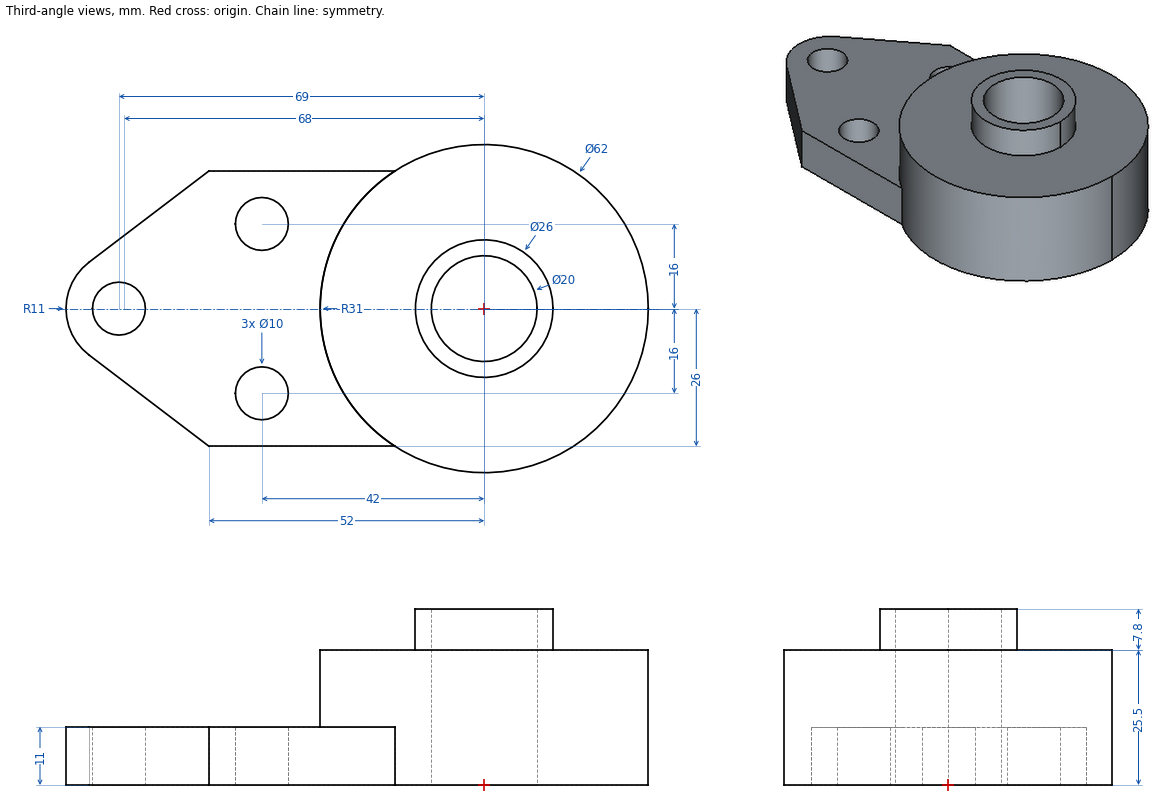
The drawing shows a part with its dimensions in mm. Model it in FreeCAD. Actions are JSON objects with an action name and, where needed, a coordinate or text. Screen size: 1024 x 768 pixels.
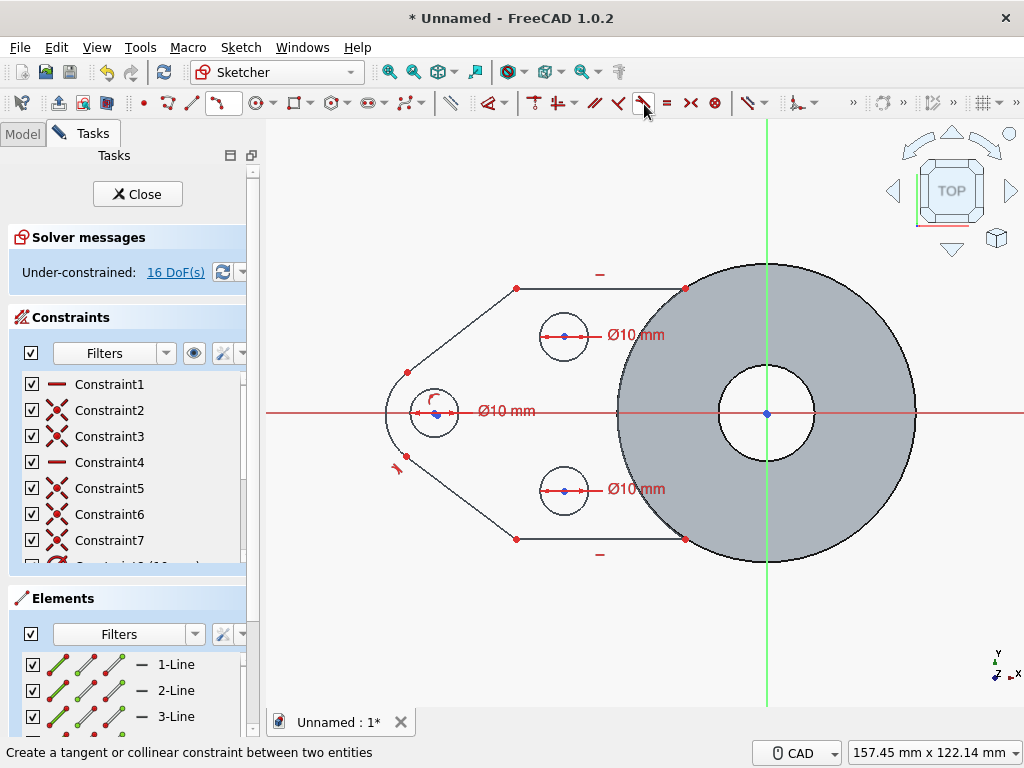
{"action": "left_click", "coordinate": [440, 348]}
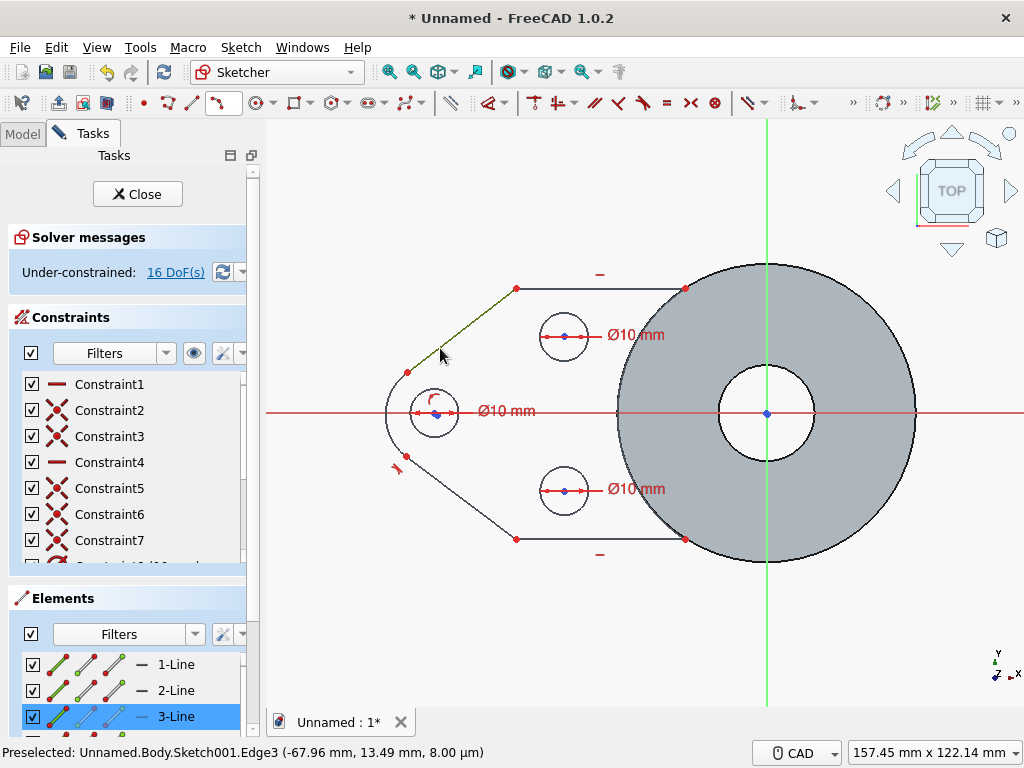
{"action": "left_click", "coordinate": [390, 395]}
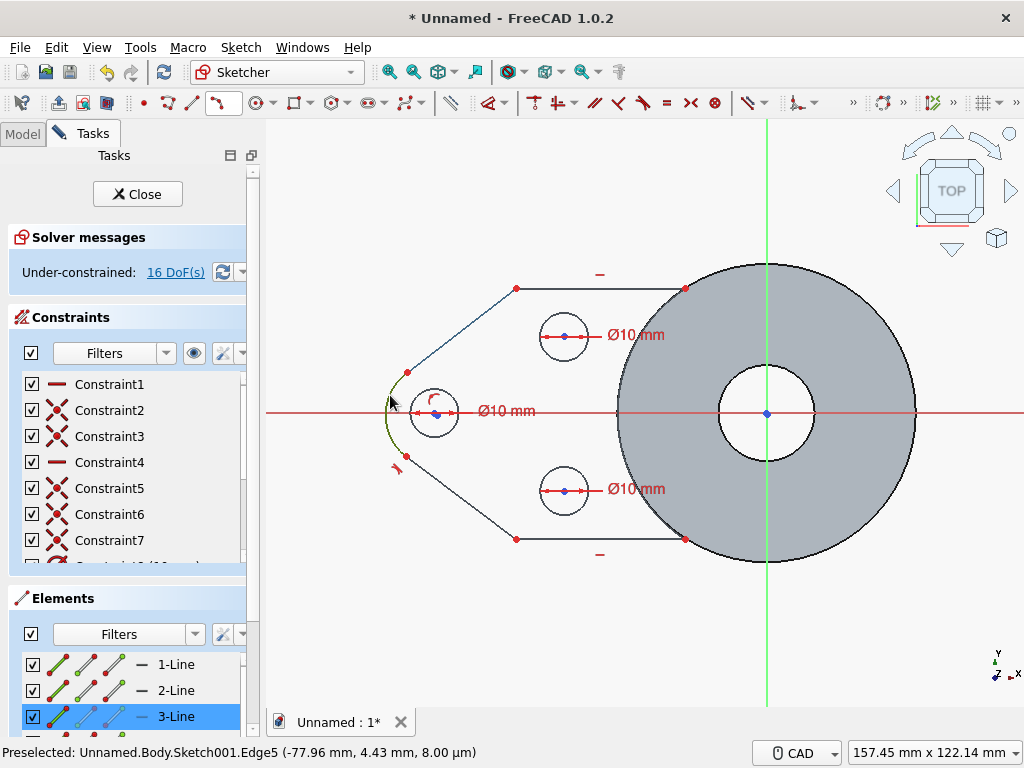
{"action": "left_click", "coordinate": [644, 104]}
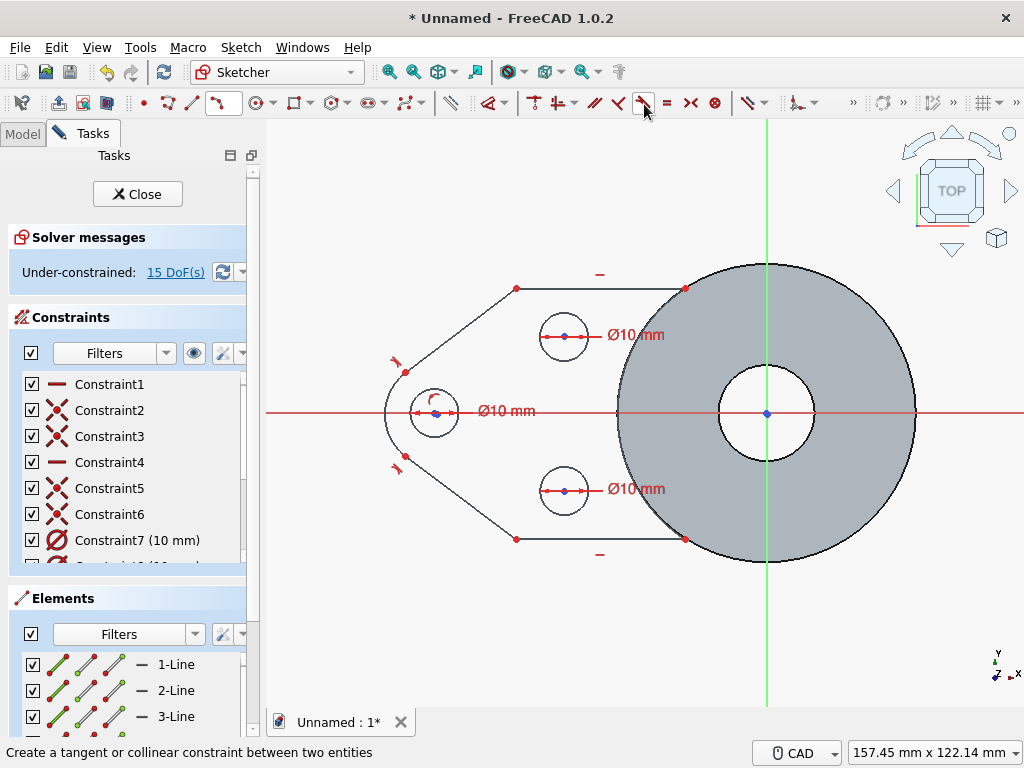
{"action": "scroll", "coordinate": [767, 414], "scroll_direction": "up", "scroll_amount": 3}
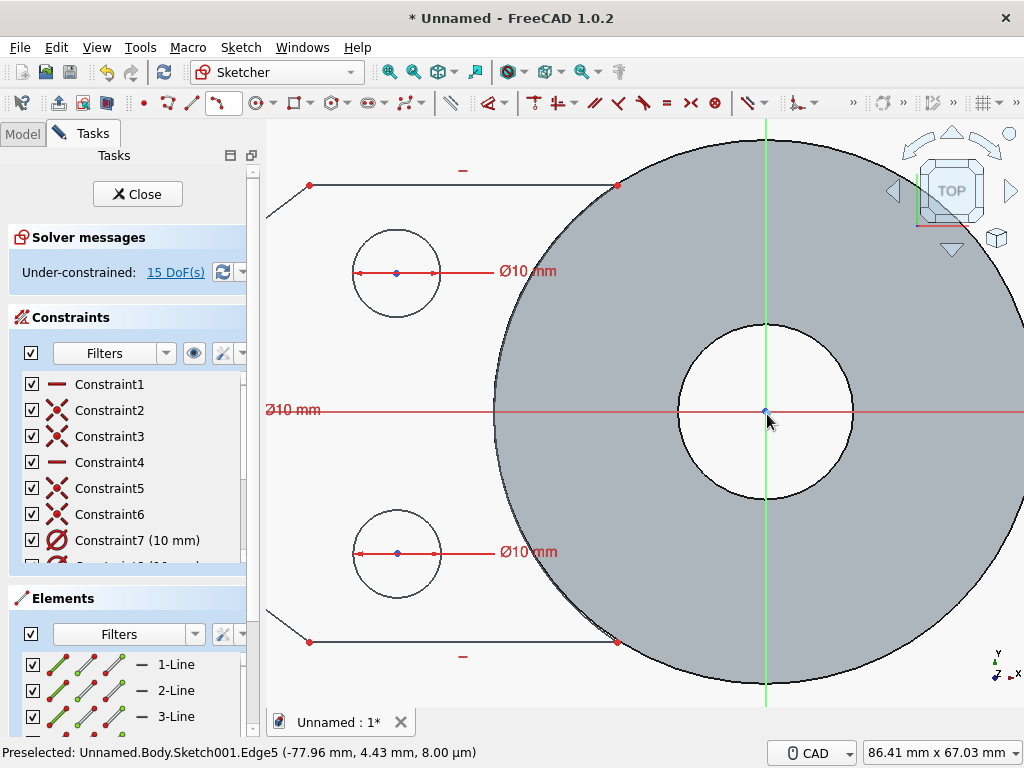
{"action": "left_click_drag", "start_coordinate": [756, 402], "coordinate": [778, 424]}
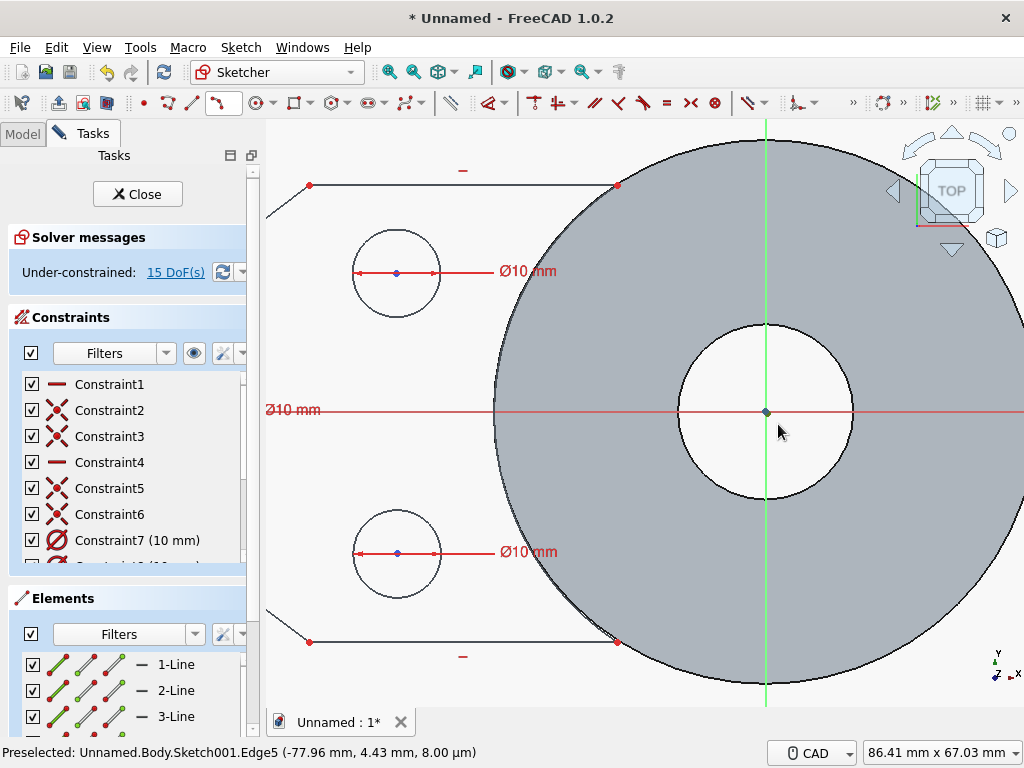
{"action": "key", "text": "c"}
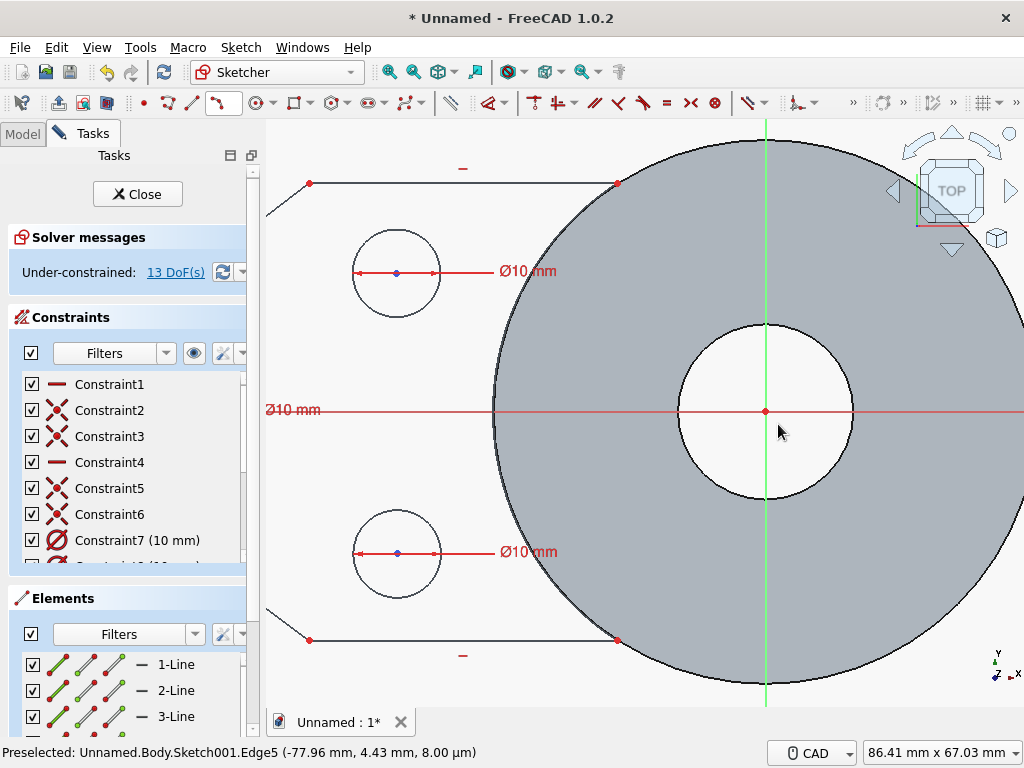
{"action": "scroll", "coordinate": [768, 414], "scroll_direction": "down", "scroll_amount": 3}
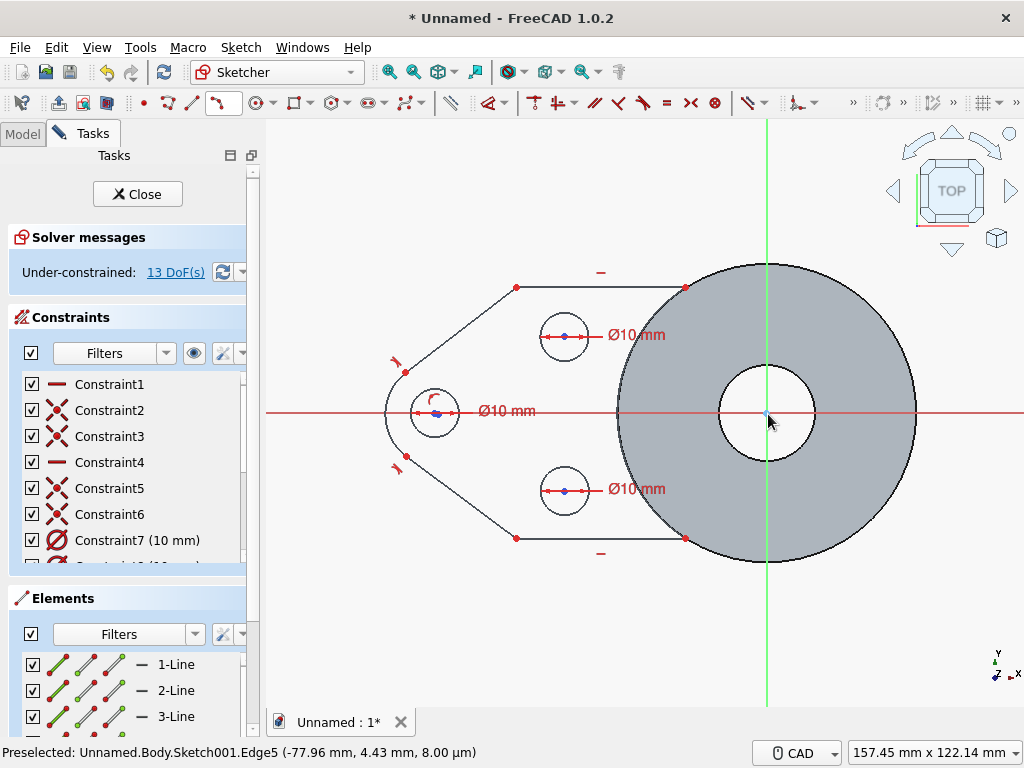
{"action": "scroll", "coordinate": [438, 414], "scroll_direction": "up", "scroll_amount": 7}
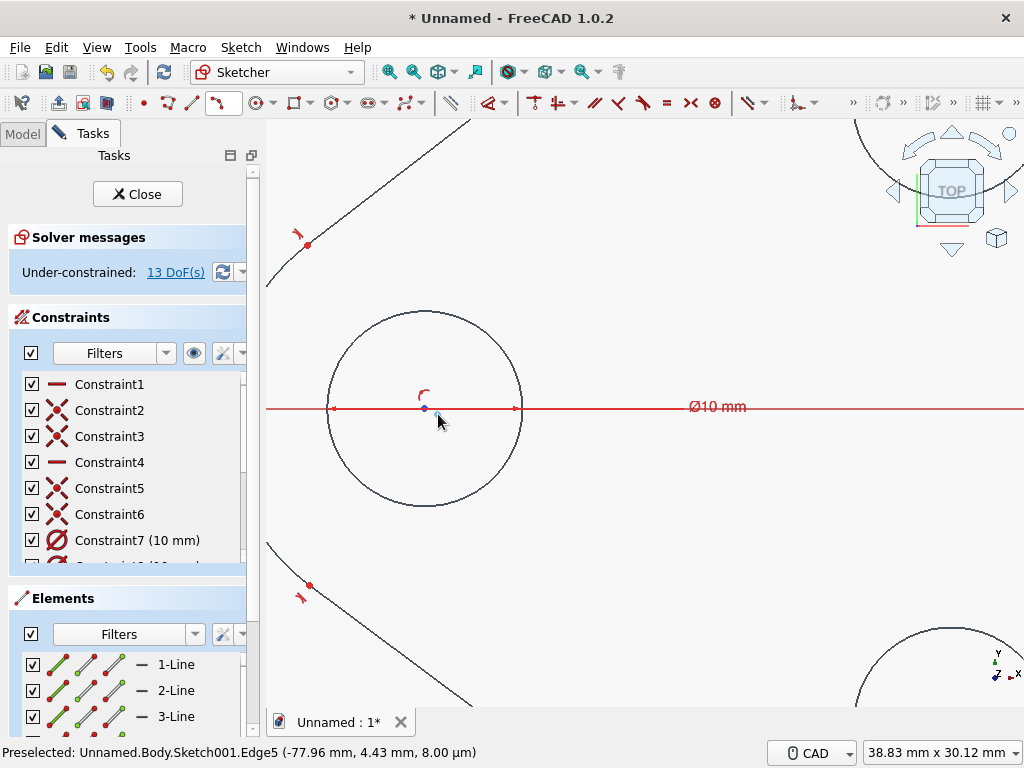
{"action": "left_click", "coordinate": [438, 414]}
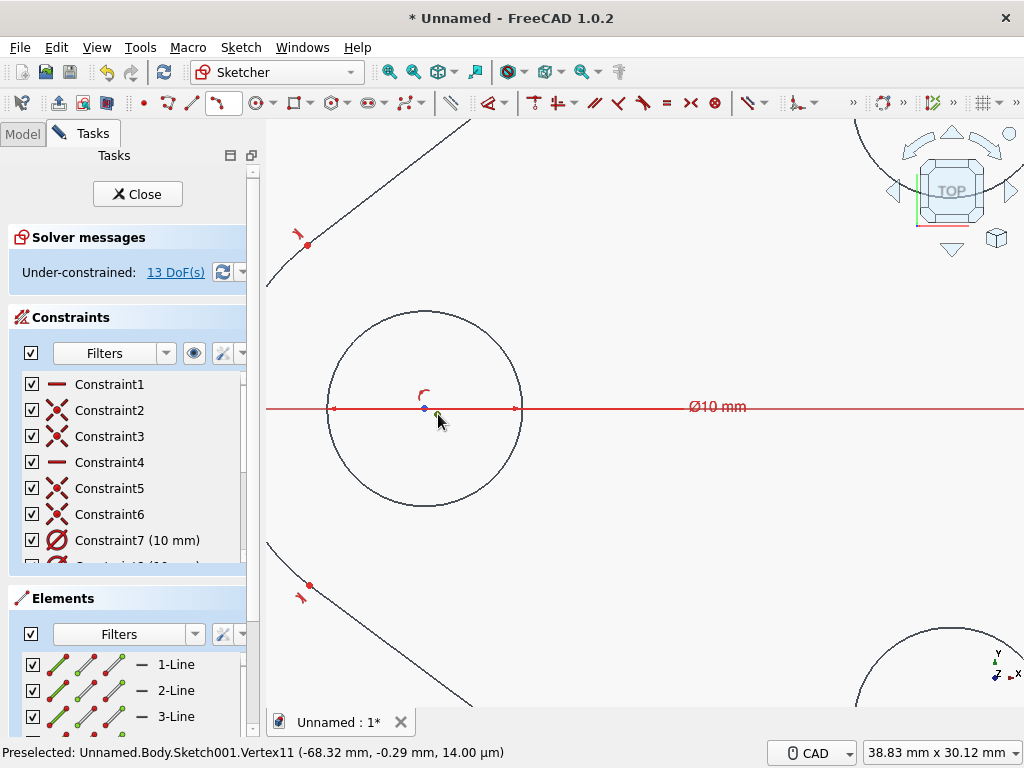
{"action": "left_click", "coordinate": [375, 409]}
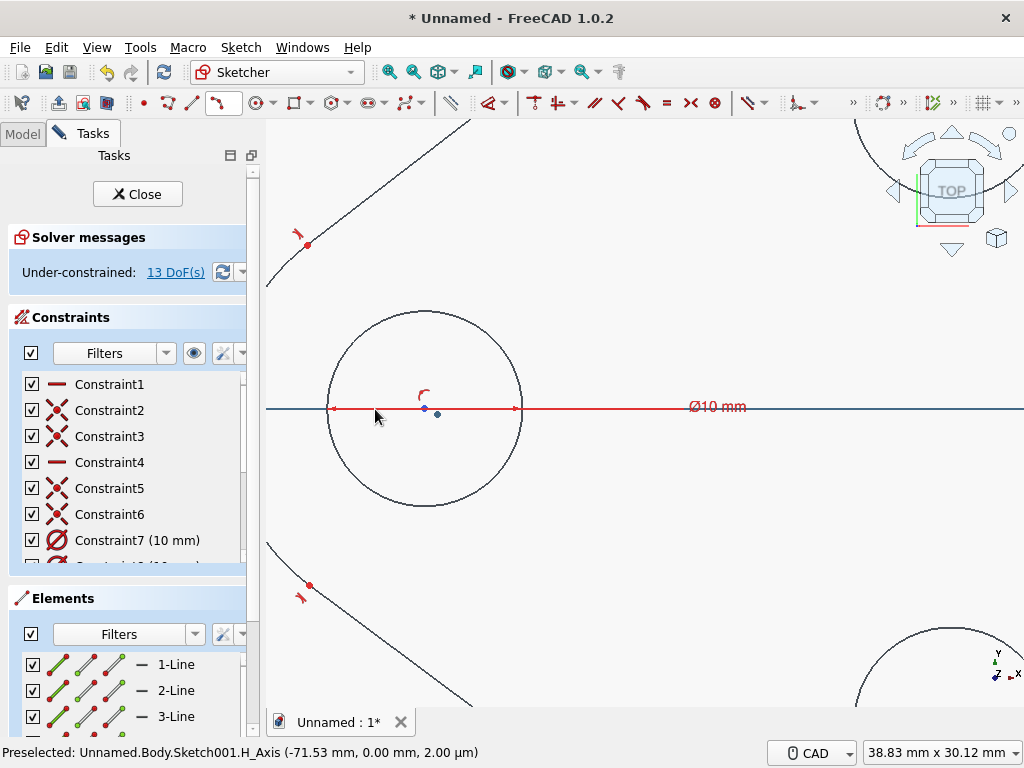
{"action": "left_click", "coordinate": [534, 104]}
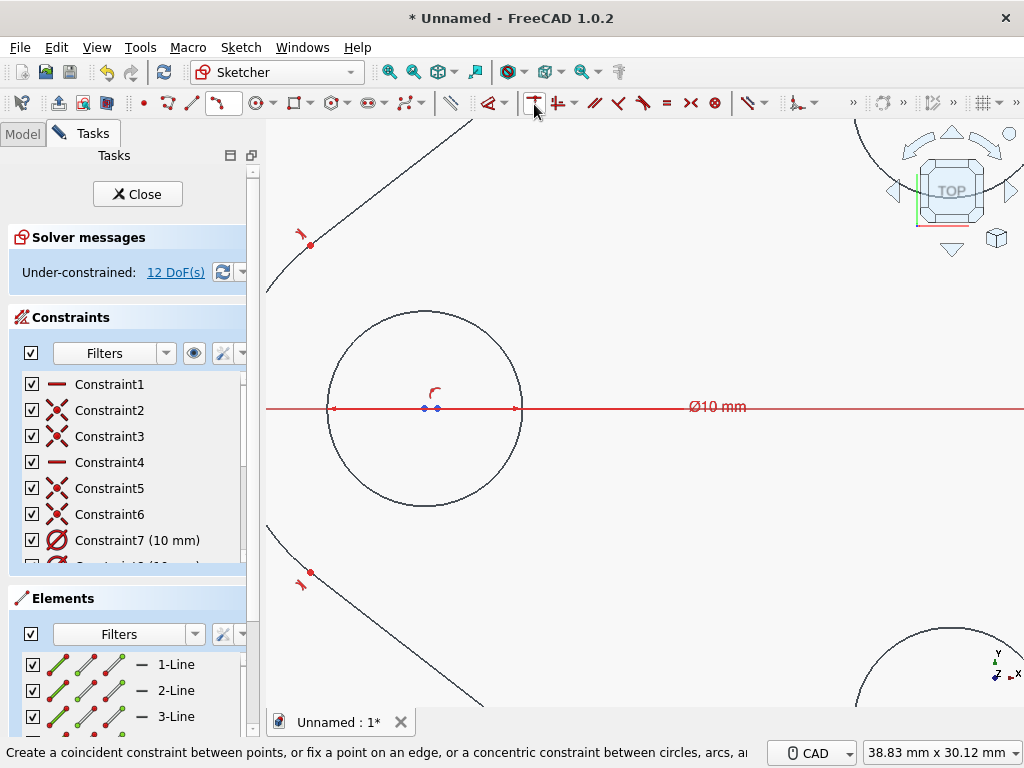
{"action": "scroll", "coordinate": [438, 414], "scroll_direction": "down", "scroll_amount": 7}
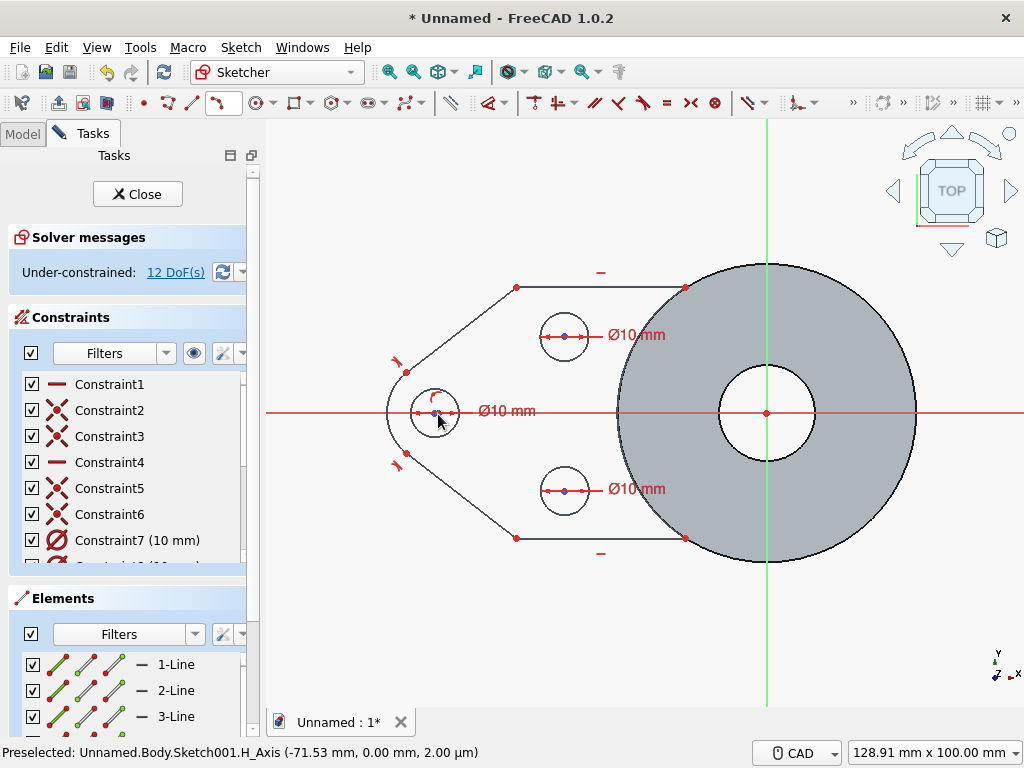
{"action": "left_click", "coordinate": [565, 491]}